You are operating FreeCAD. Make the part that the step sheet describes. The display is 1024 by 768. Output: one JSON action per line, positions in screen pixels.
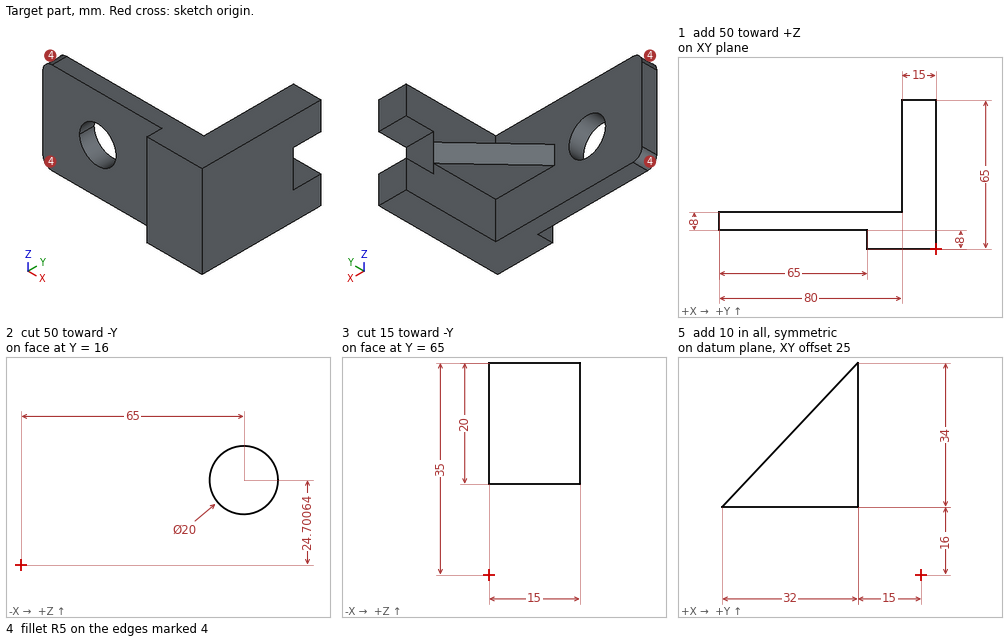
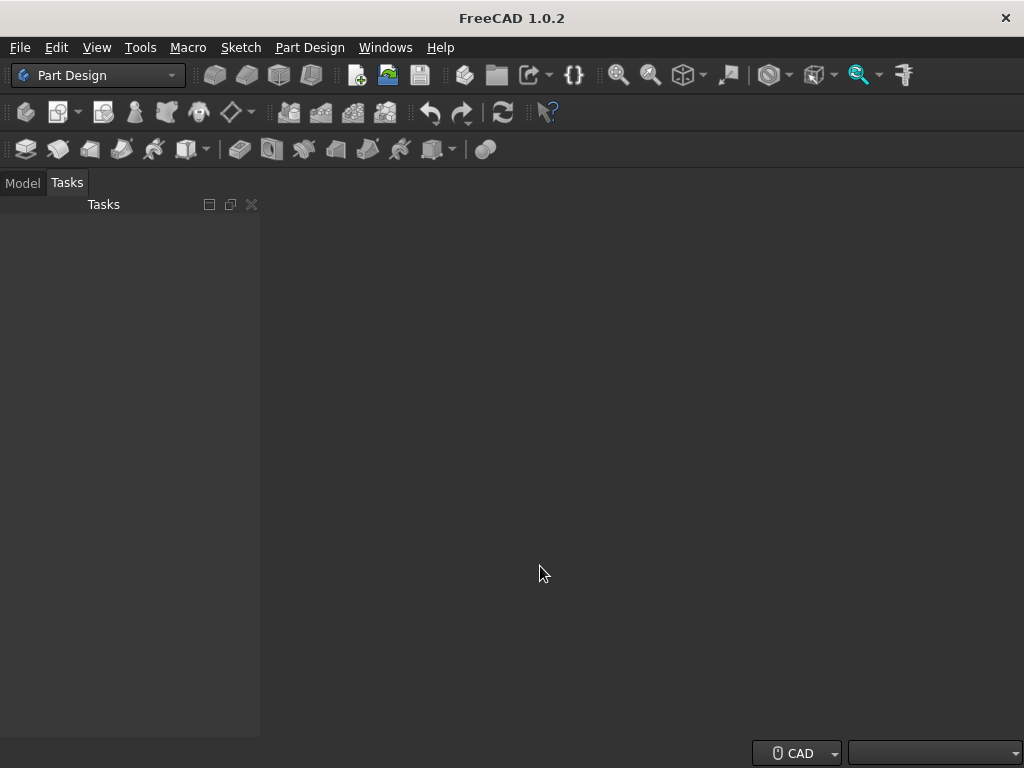
{"action": "left_click", "coordinate": [356, 76]}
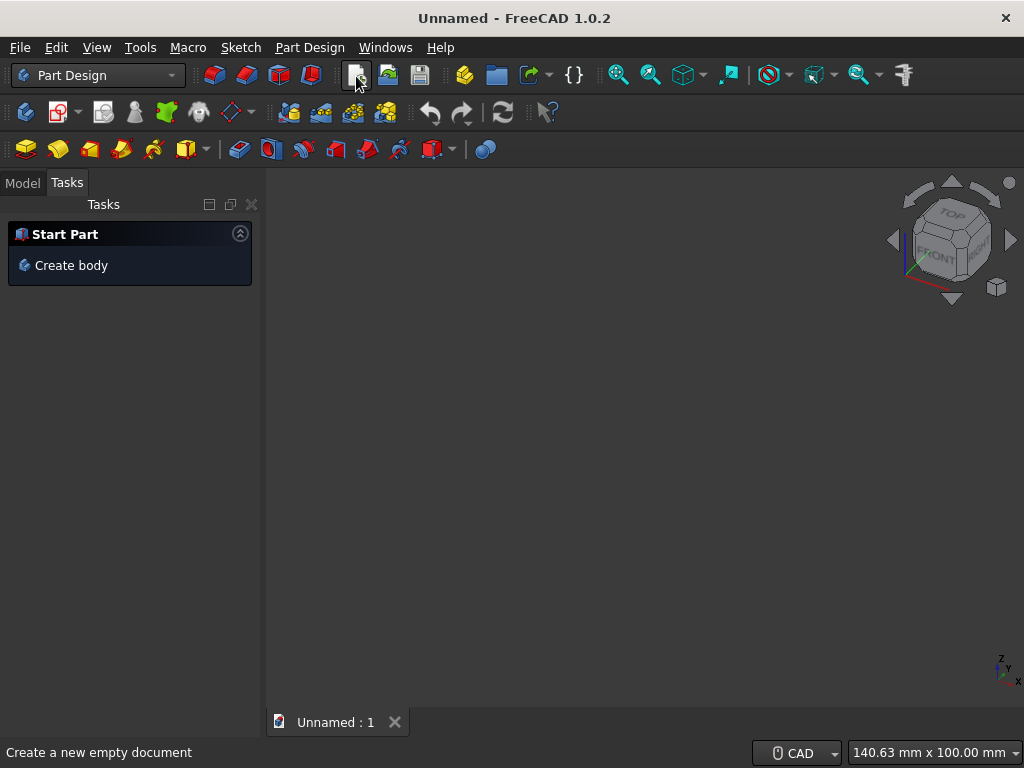
{"action": "left_click", "coordinate": [58, 112]}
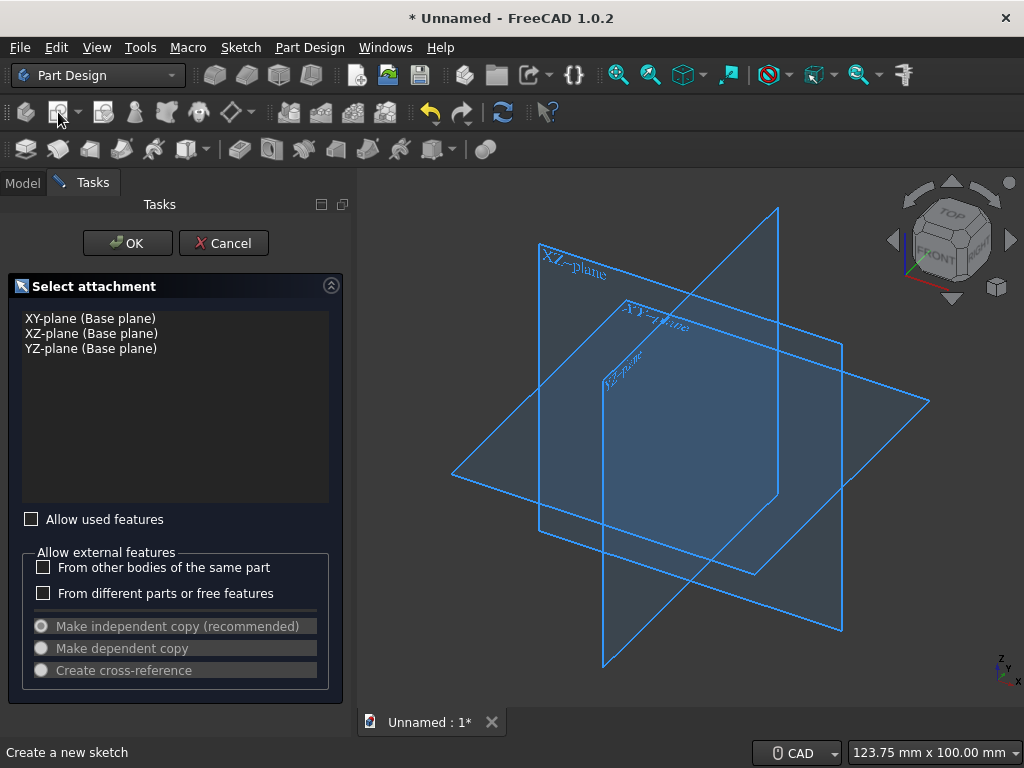
{"action": "left_click", "coordinate": [82, 318]}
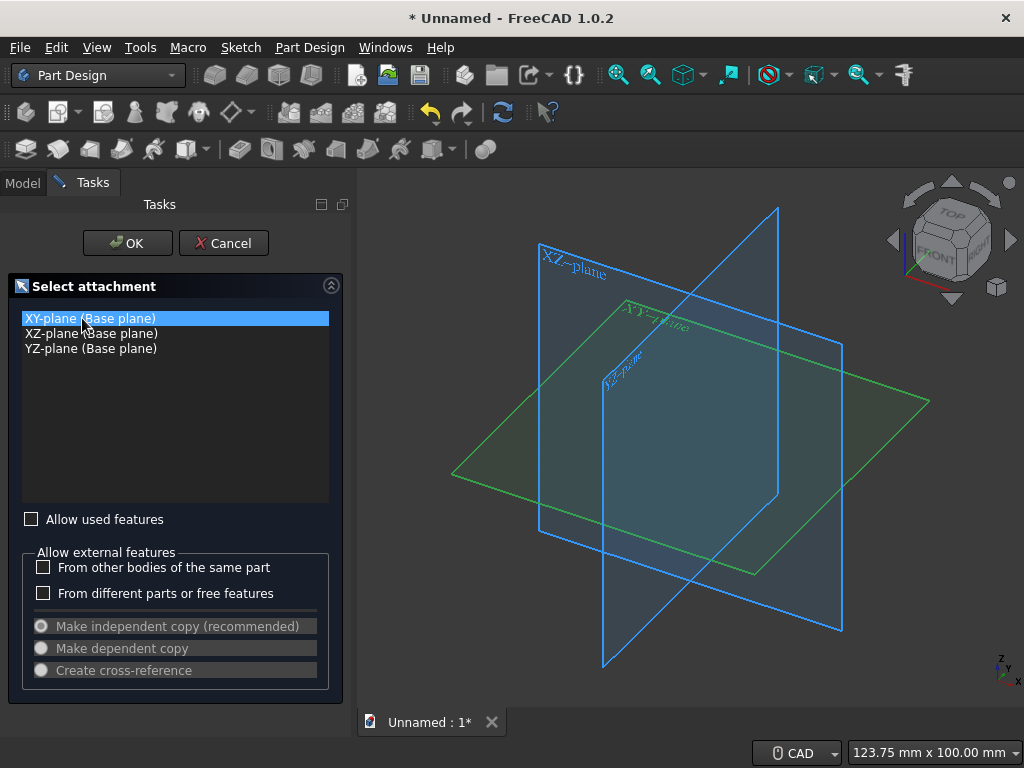
{"action": "left_click", "coordinate": [128, 243]}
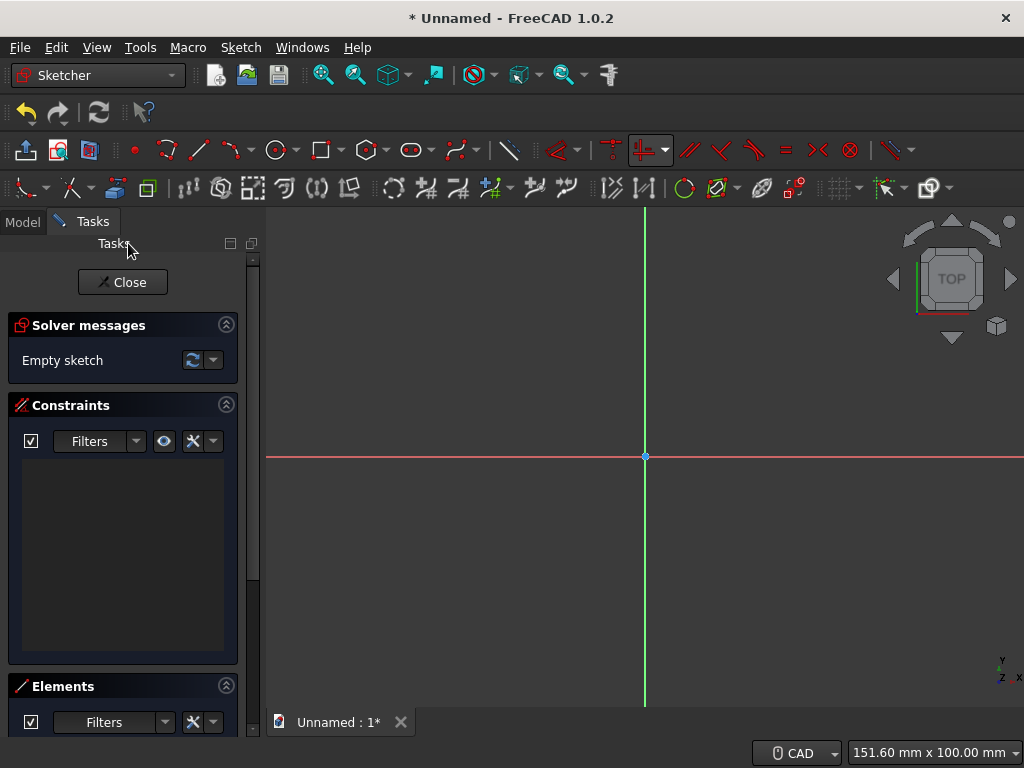
{"action": "scroll", "coordinate": [859, 679], "scroll_direction": "down", "scroll_amount": 2}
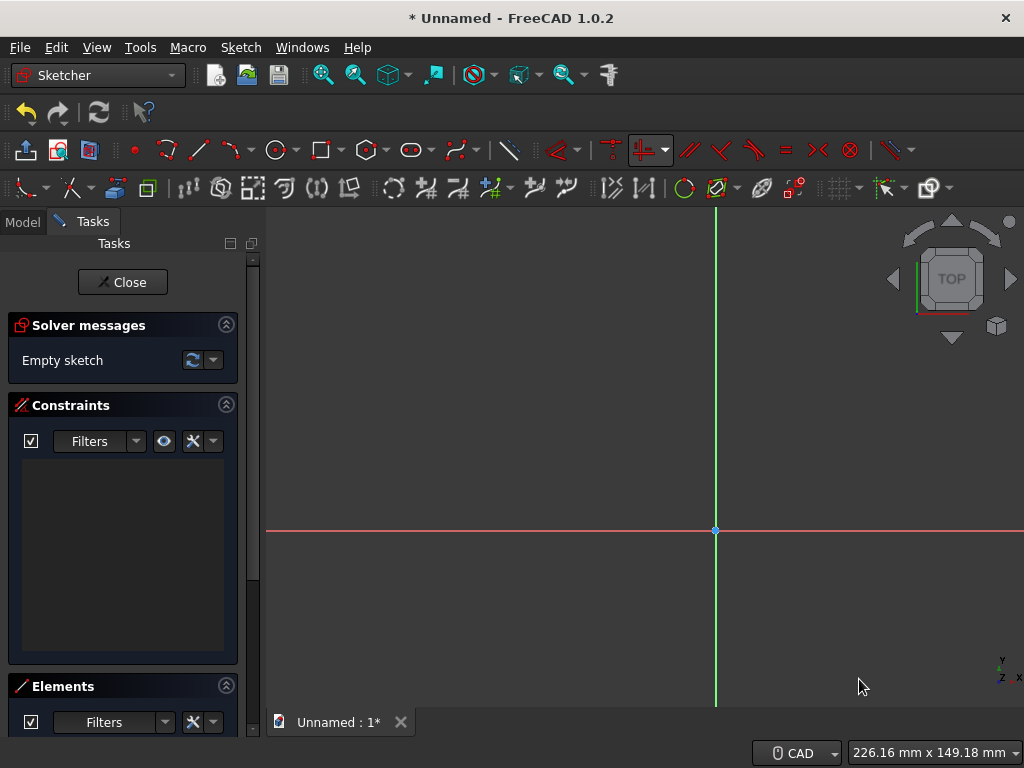
{"action": "left_click", "coordinate": [168, 150]}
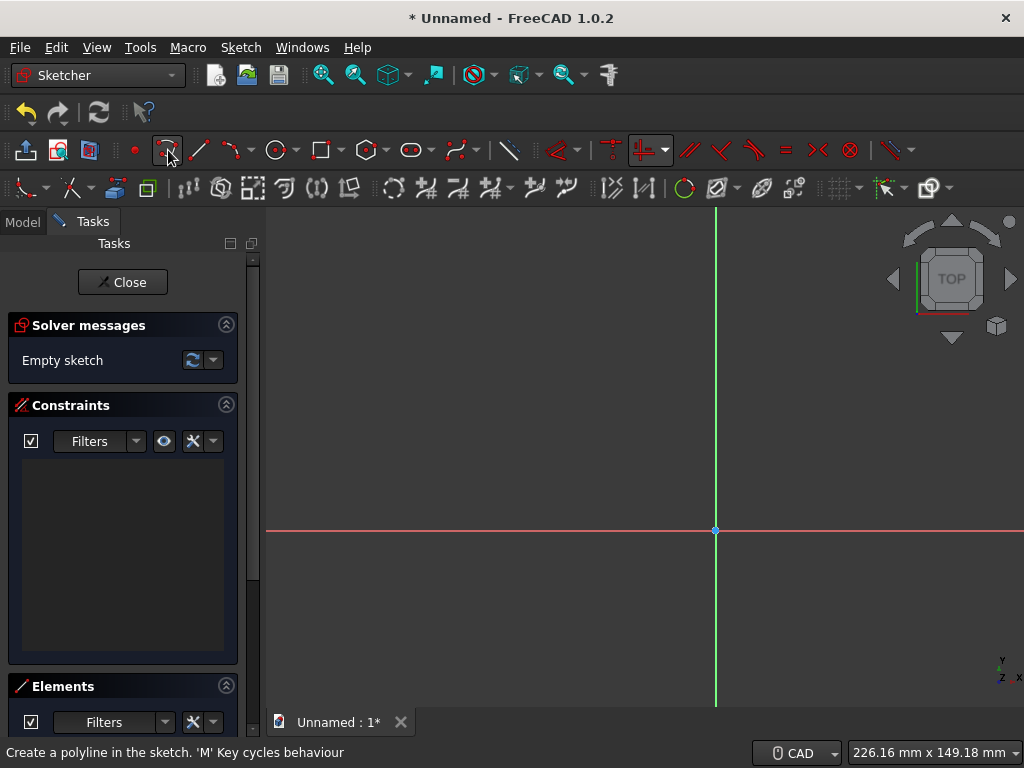
{"action": "left_click", "coordinate": [716, 531]}
{"action": "left_click", "coordinate": [707, 313]}
{"action": "left_click", "coordinate": [666, 313]}
{"action": "left_click", "coordinate": [666, 477]}
{"action": "left_click", "coordinate": [397, 477]}
{"action": "left_click", "coordinate": [397, 504]}
{"action": "left_click", "coordinate": [615, 504]}
{"action": "left_click", "coordinate": [615, 522]}
{"action": "left_click", "coordinate": [716, 531]}
{"action": "key", "text": "Escape"}
{"action": "key", "text": "Escape"}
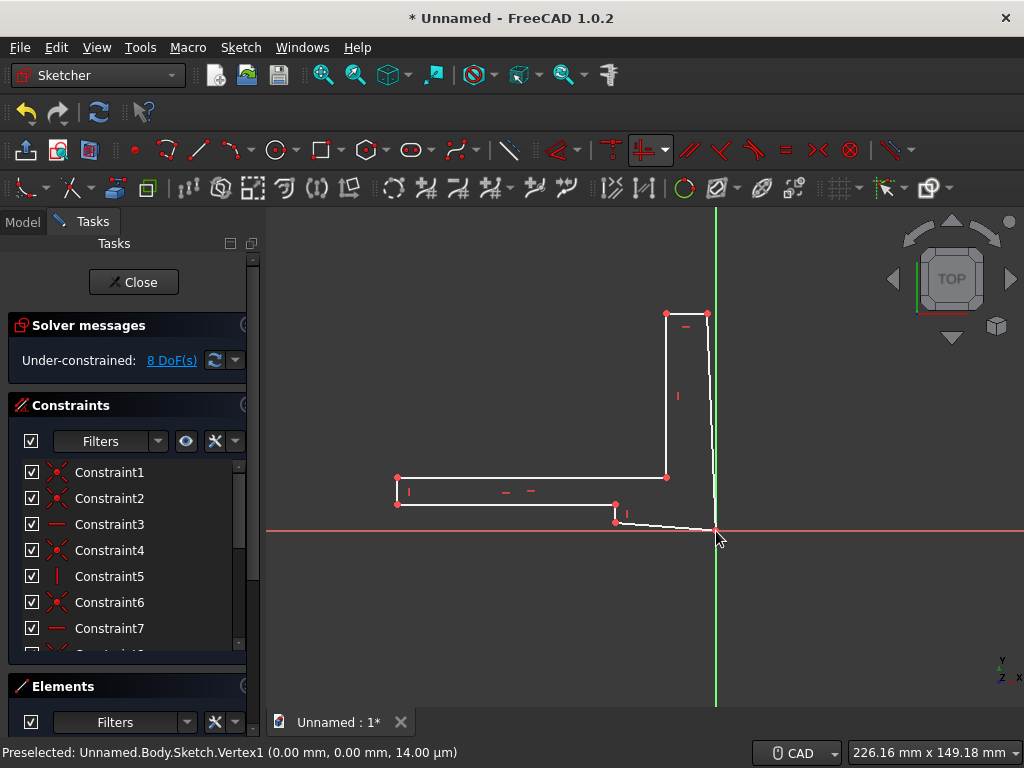
{"action": "left_click", "coordinate": [713, 466]}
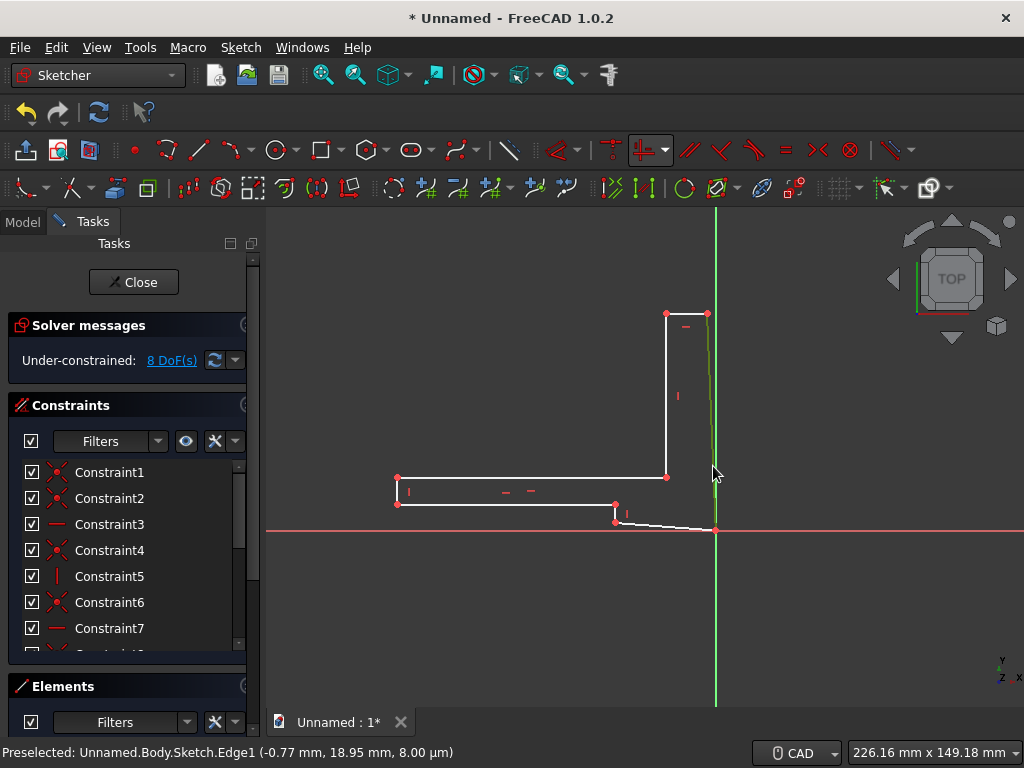
{"action": "key", "text": "v"}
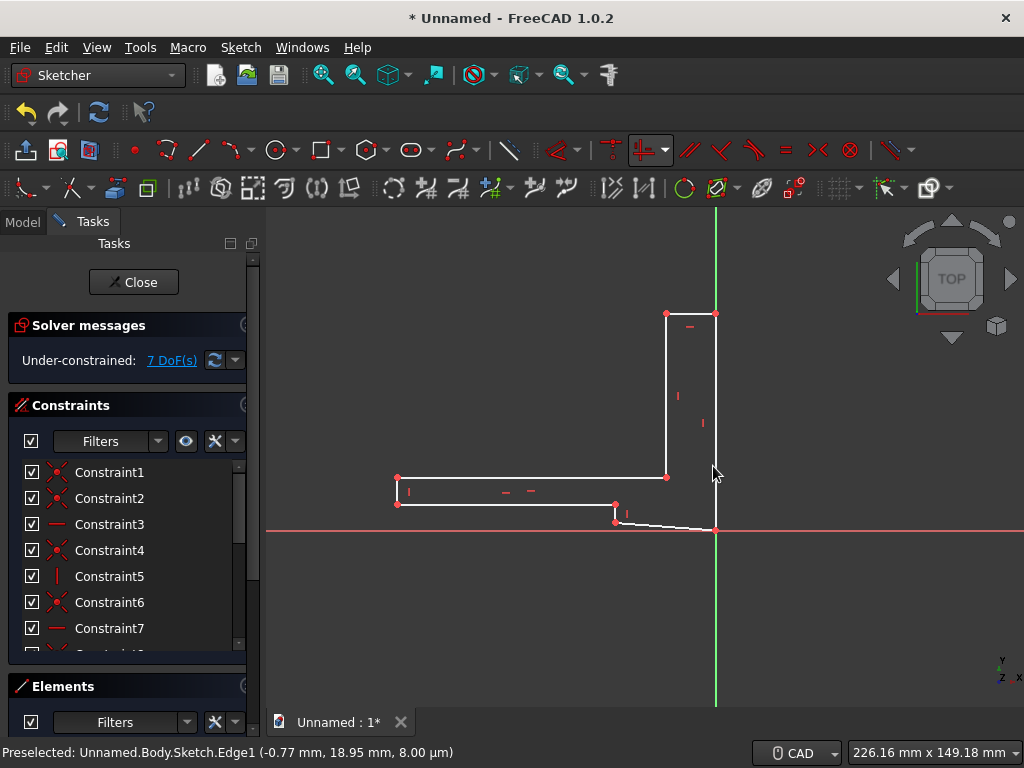
{"action": "left_click", "coordinate": [686, 528]}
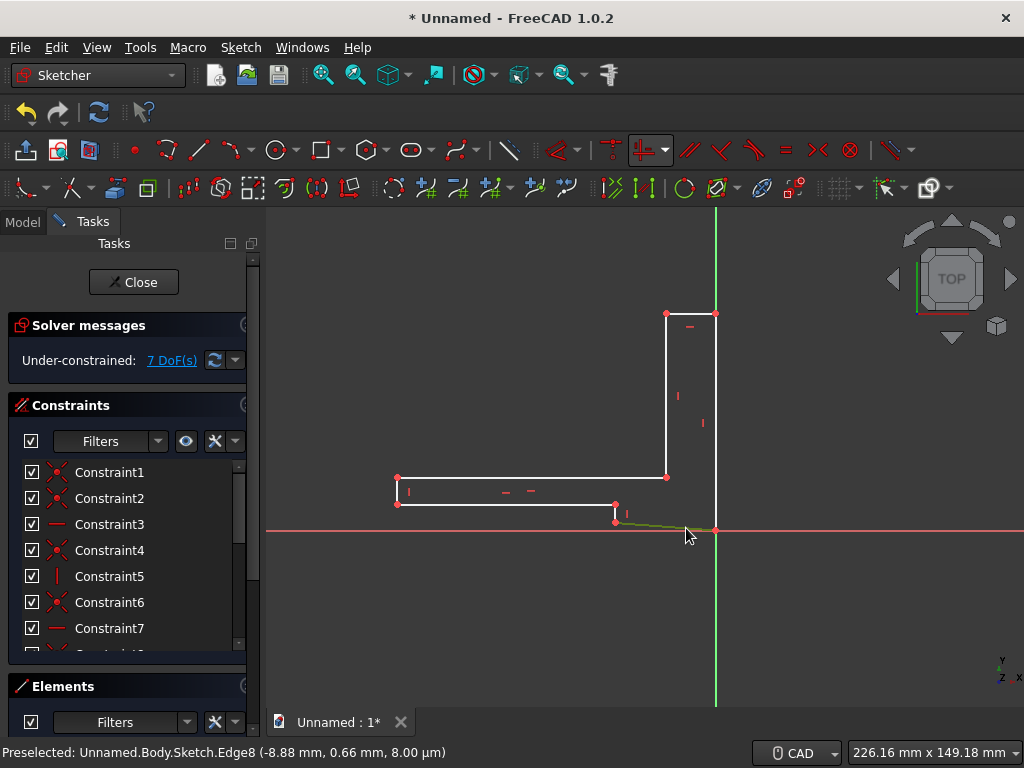
{"action": "left_click", "coordinate": [668, 150]}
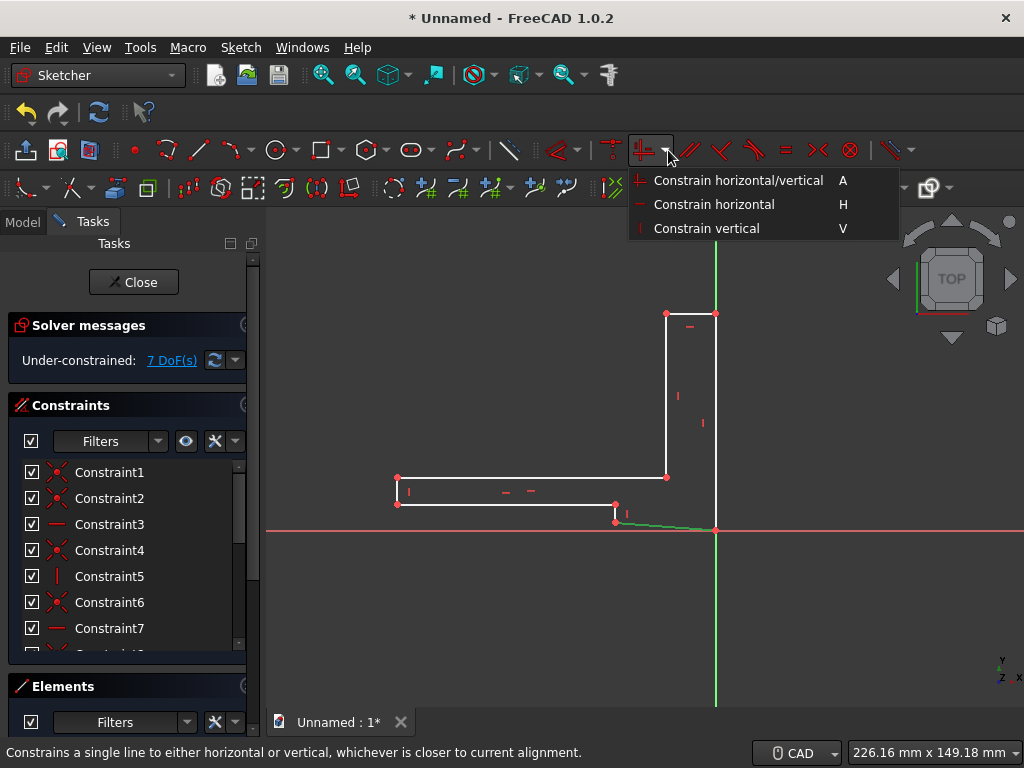
{"action": "left_click", "coordinate": [764, 204]}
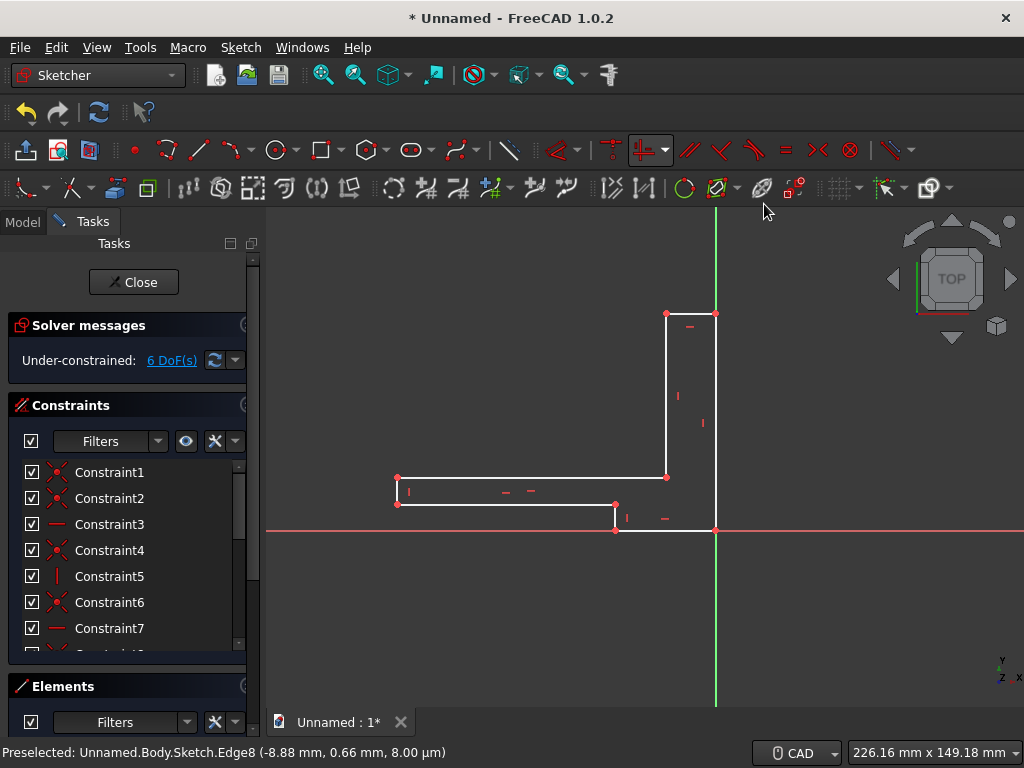
{"action": "left_click", "coordinate": [556, 150]}